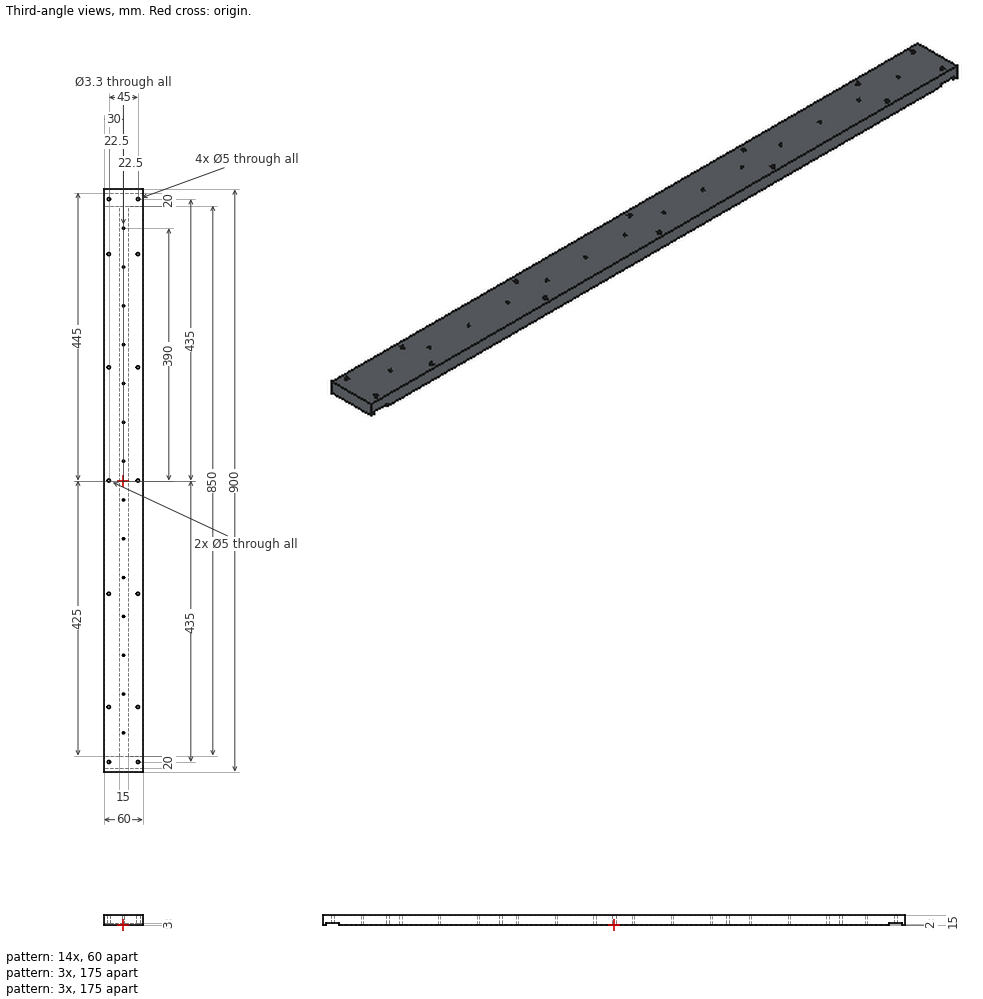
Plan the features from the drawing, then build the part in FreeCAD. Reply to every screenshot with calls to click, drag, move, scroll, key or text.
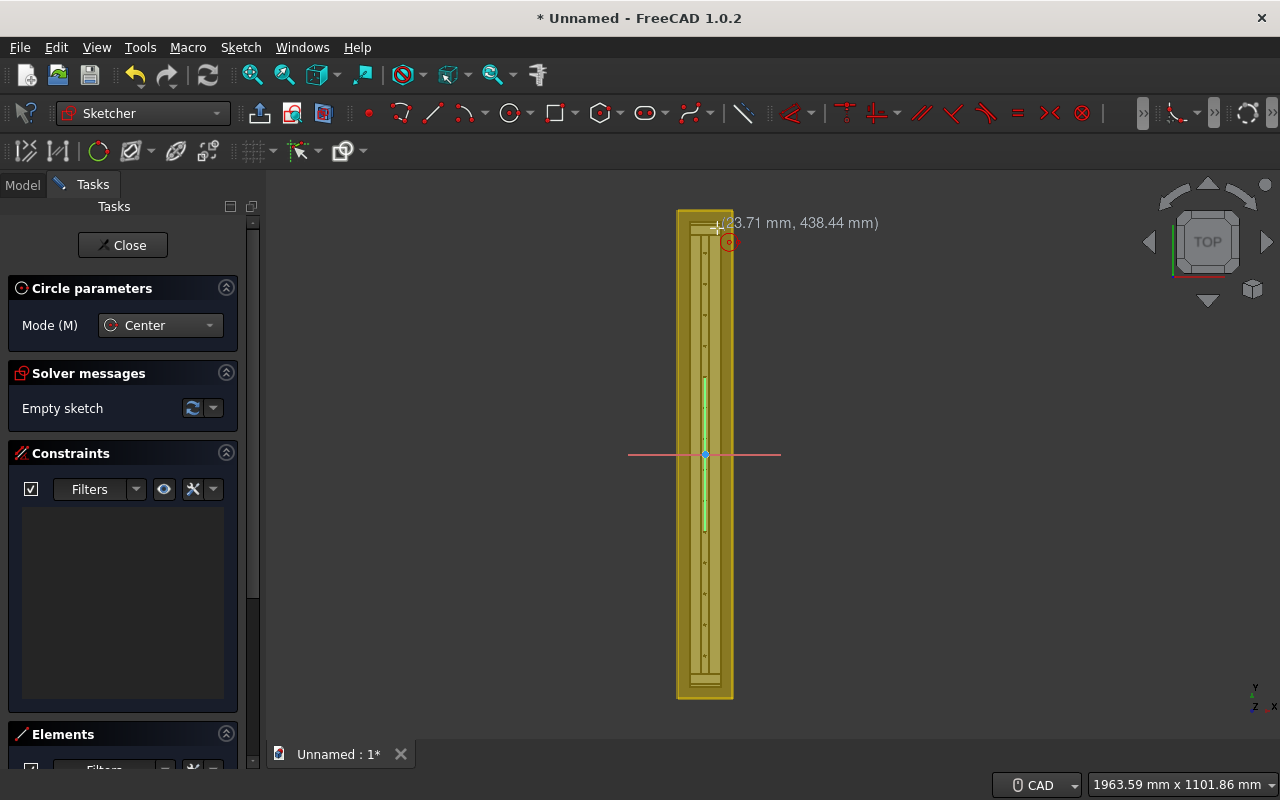
scroll(717, 230, up, 2)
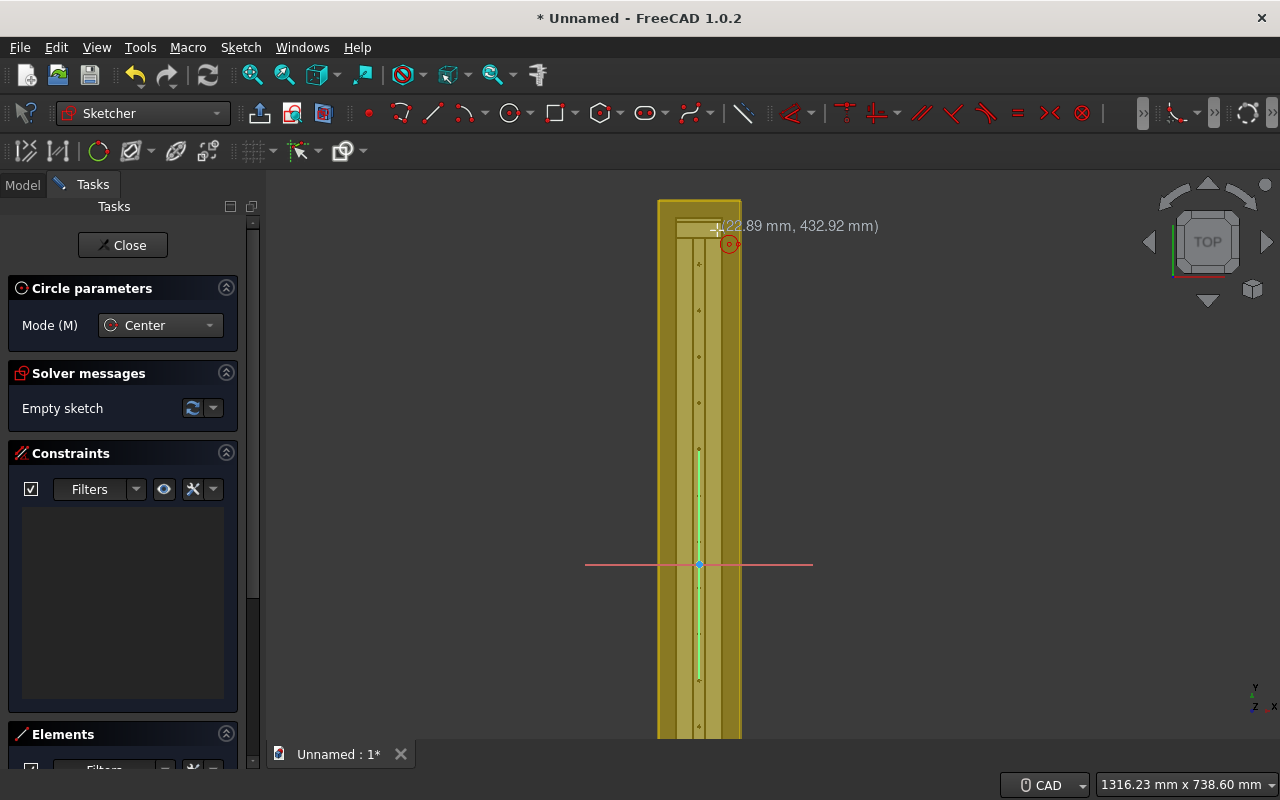
click(716, 230)
move(718, 228)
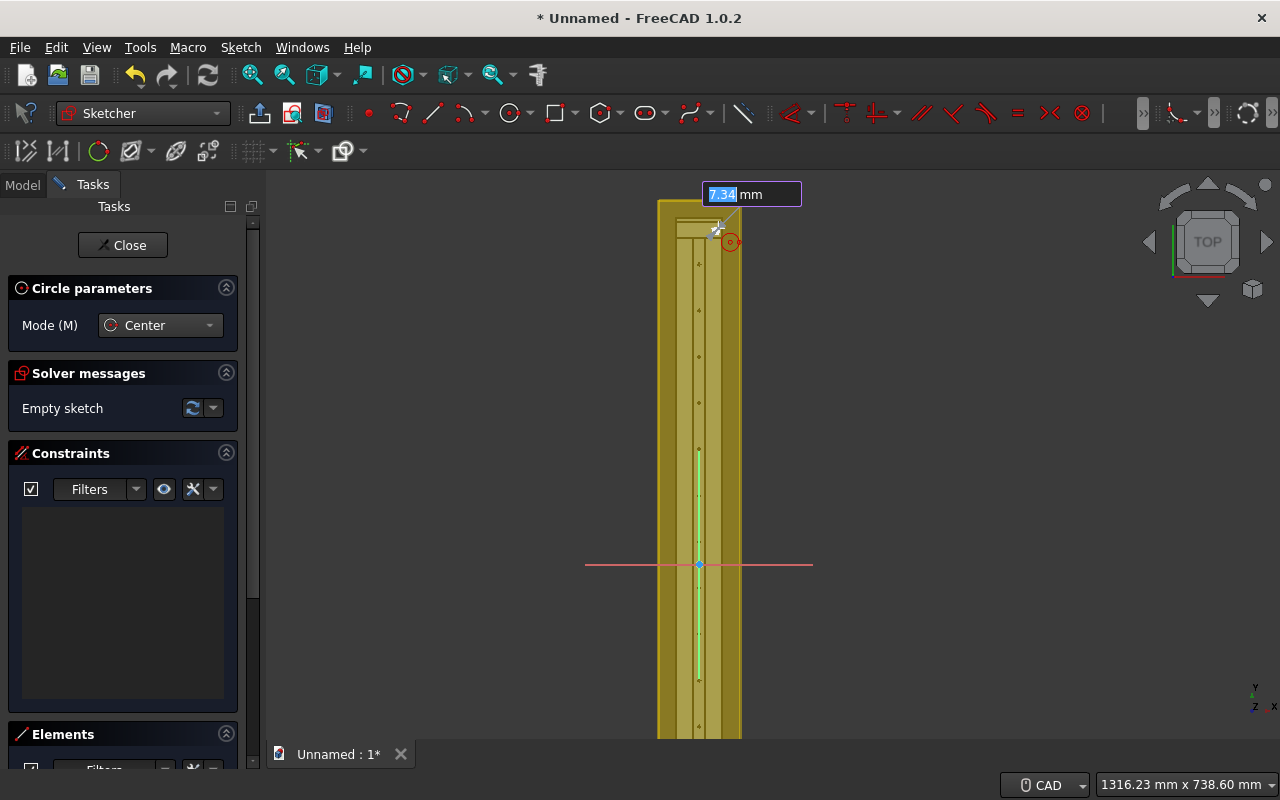
text(5)
key(Return)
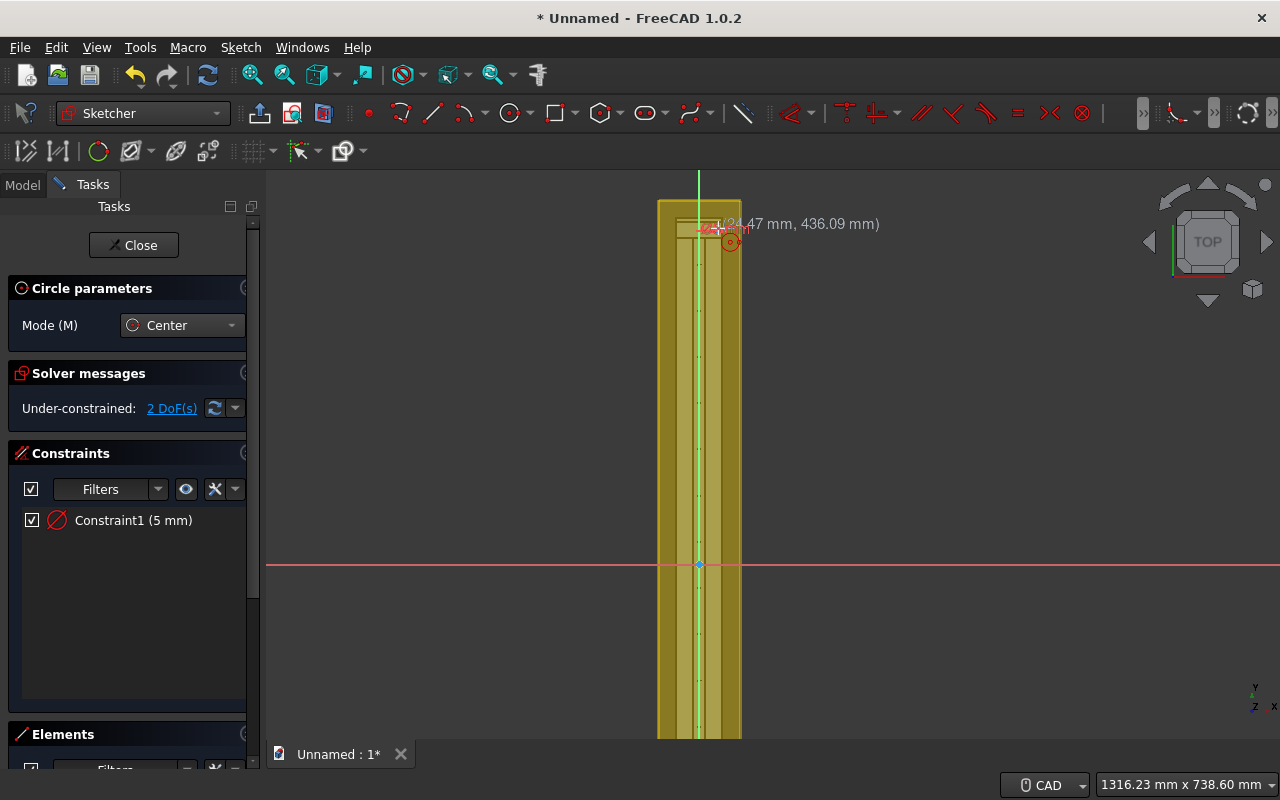
scroll(682, 230, up, 13)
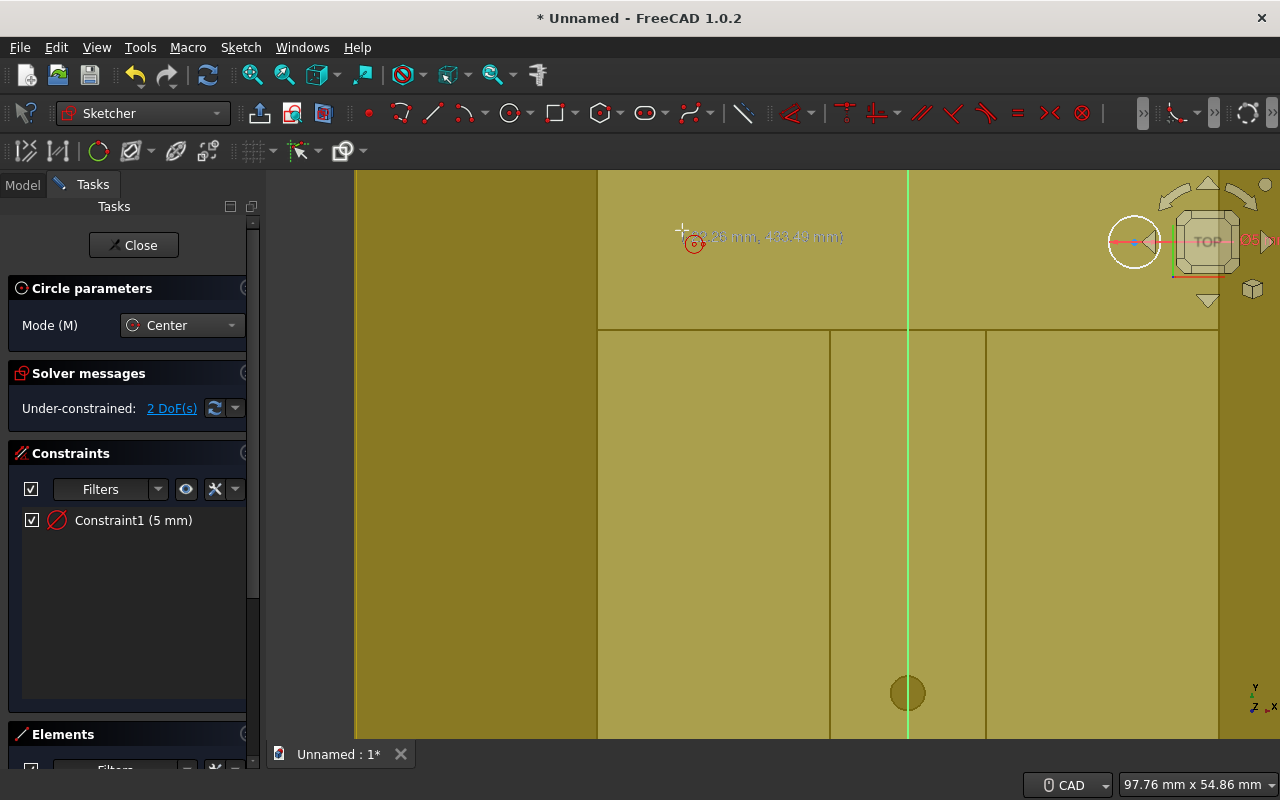
scroll(694, 230, down, 15)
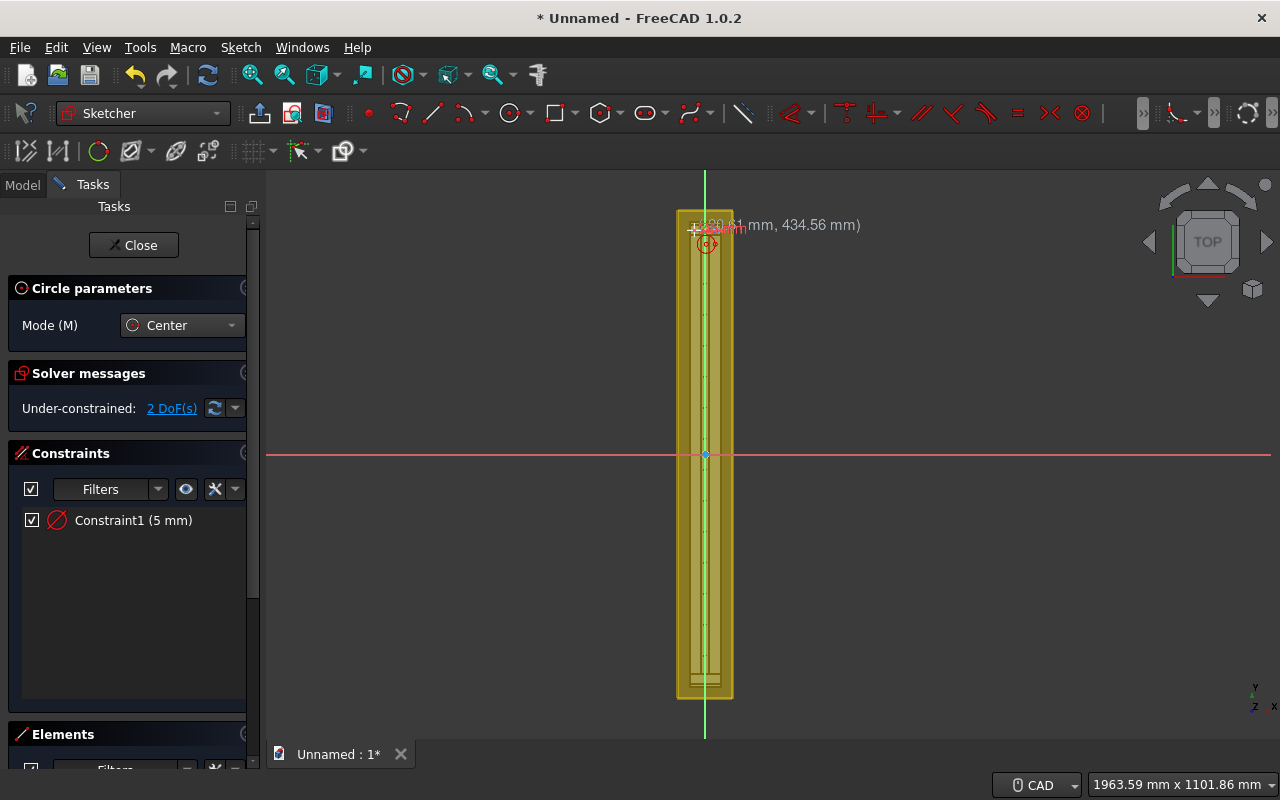
scroll(693, 230, up, 2)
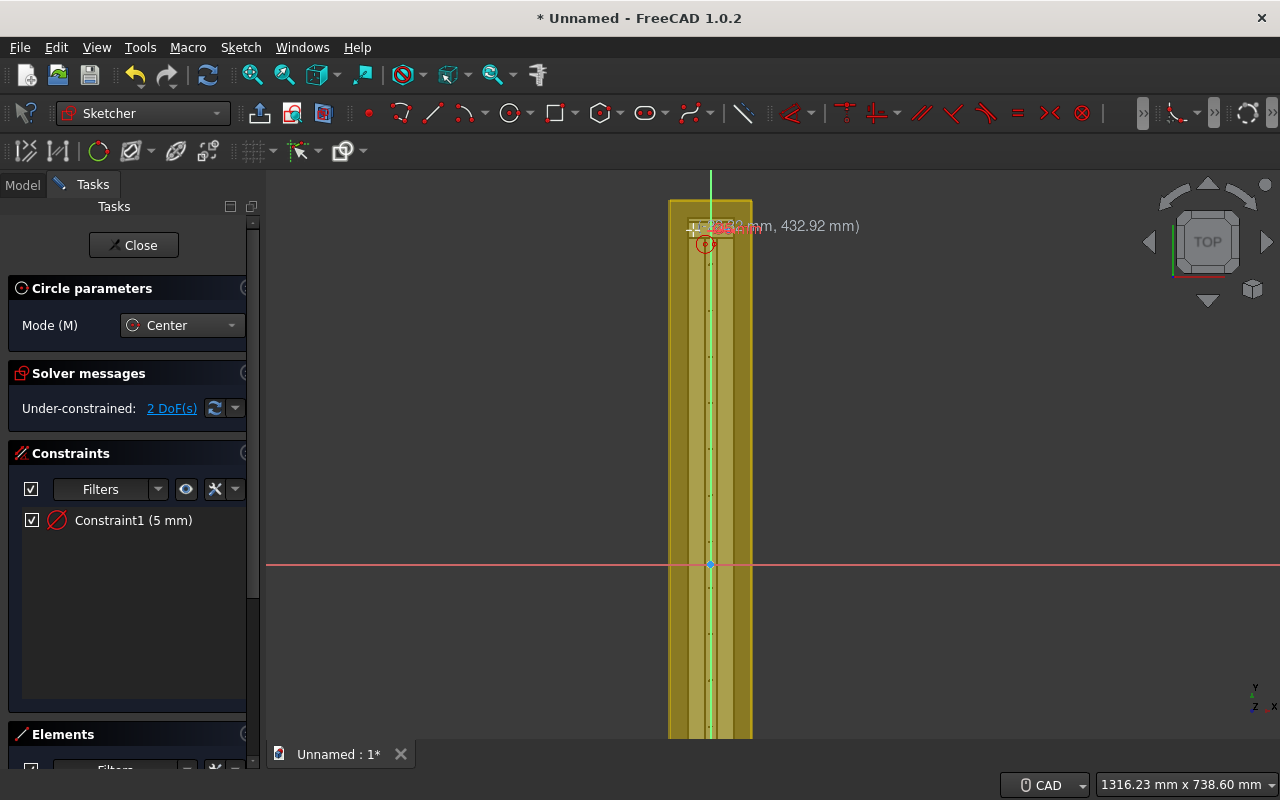
click(693, 230)
move(695, 228)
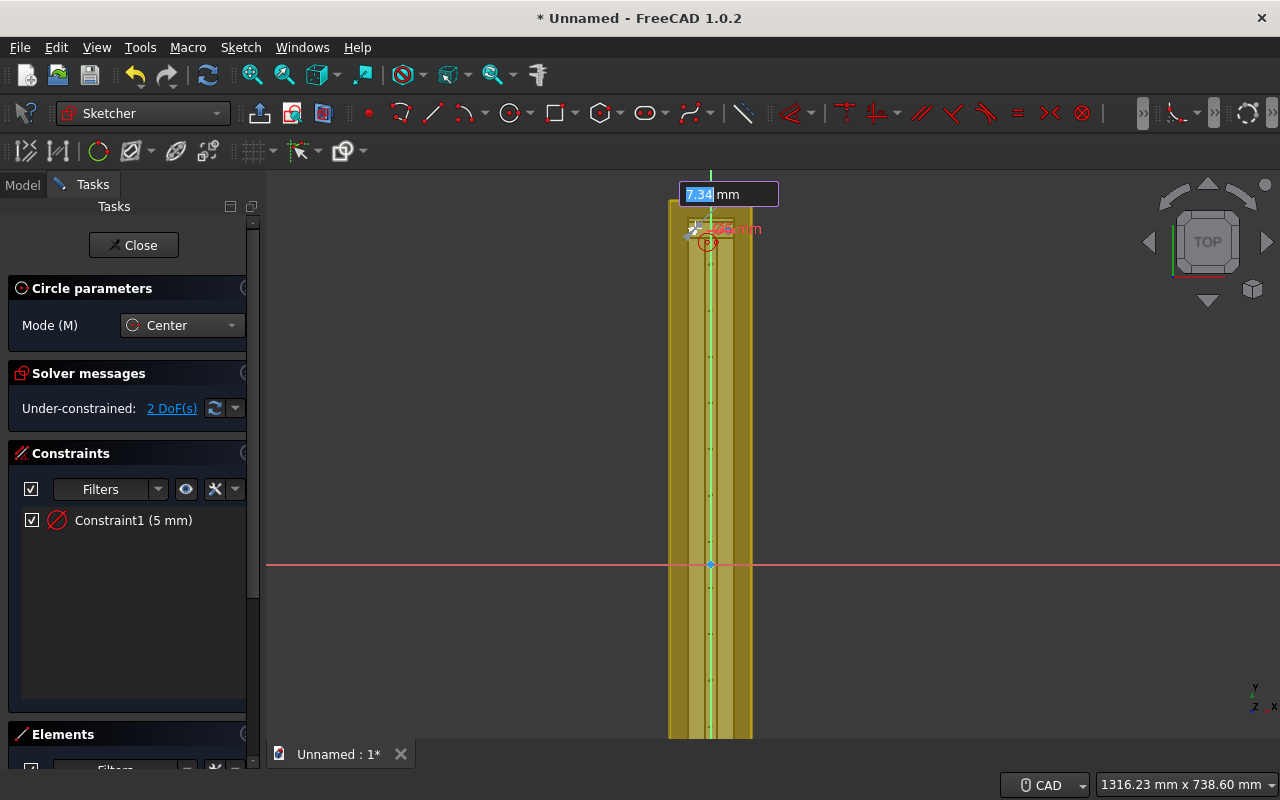
text(5)
key(Return)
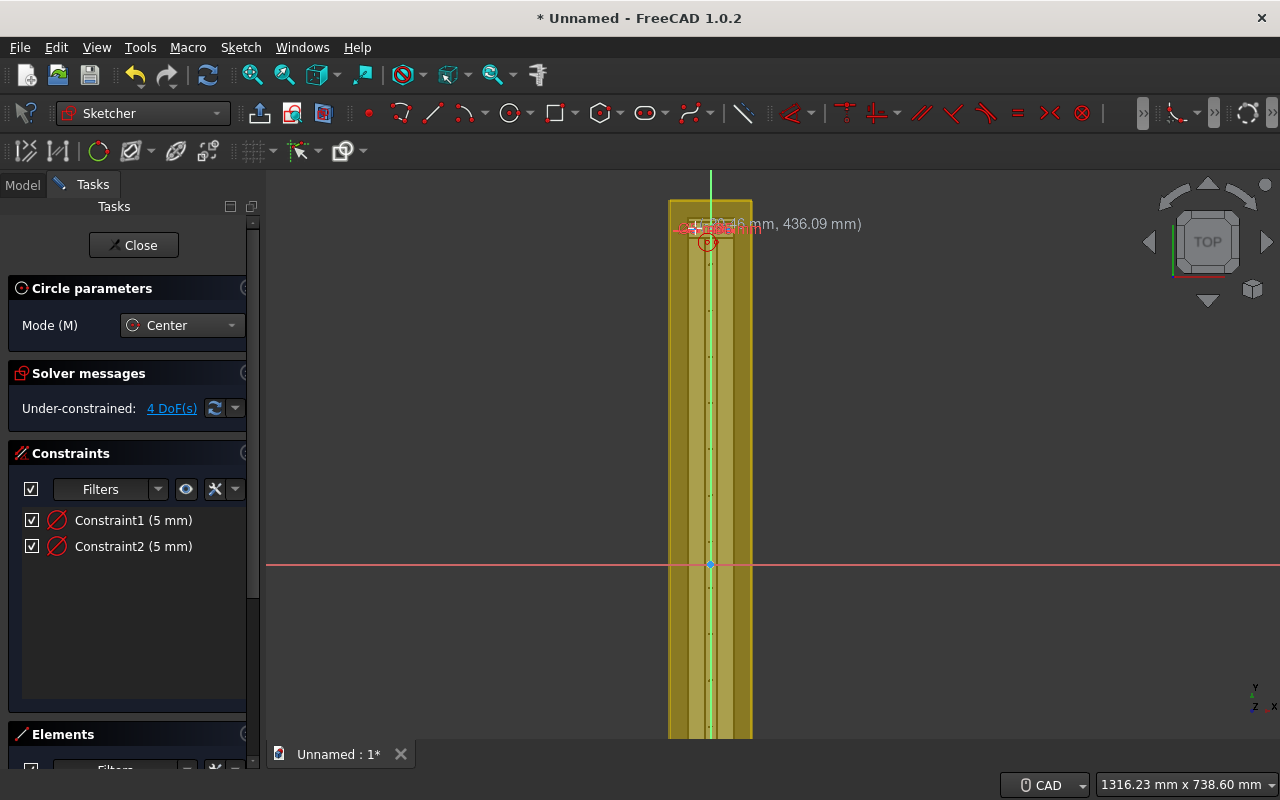
scroll(697, 320, down, 3)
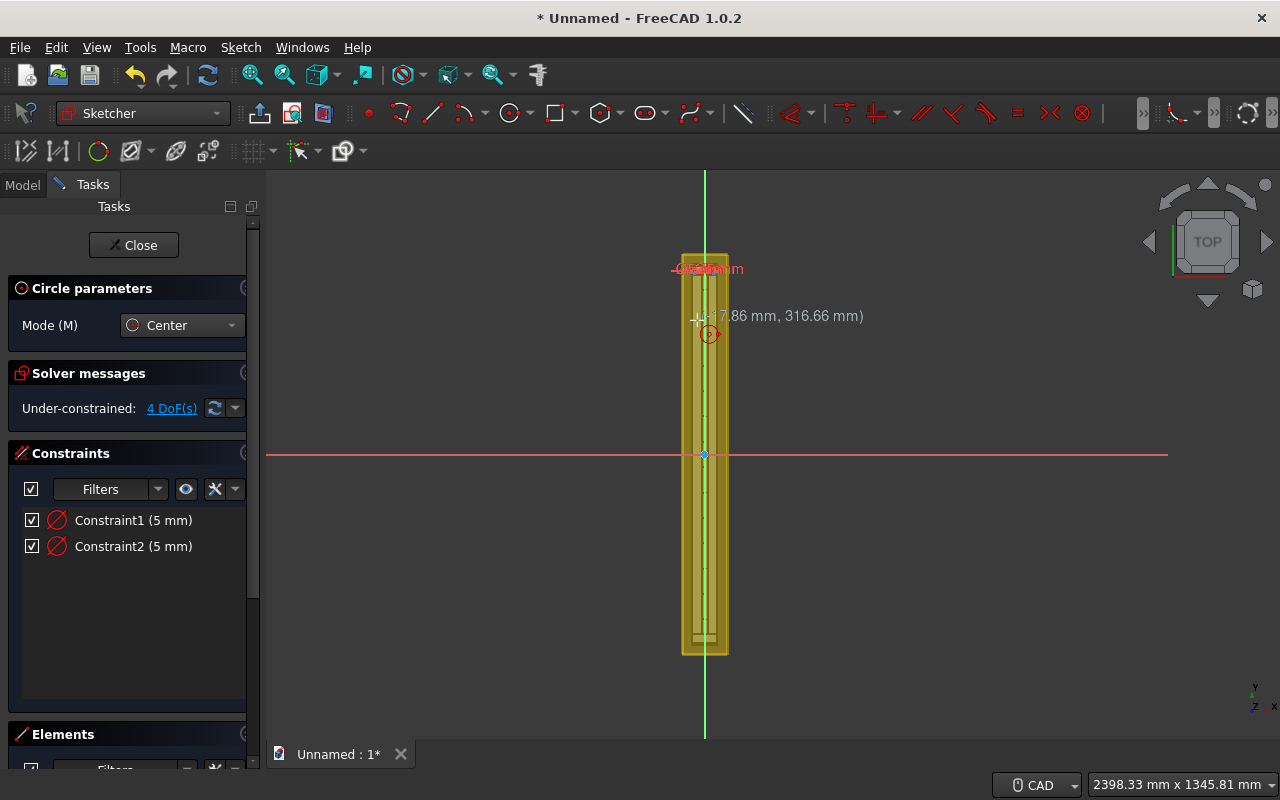
scroll(714, 638, up, 16)